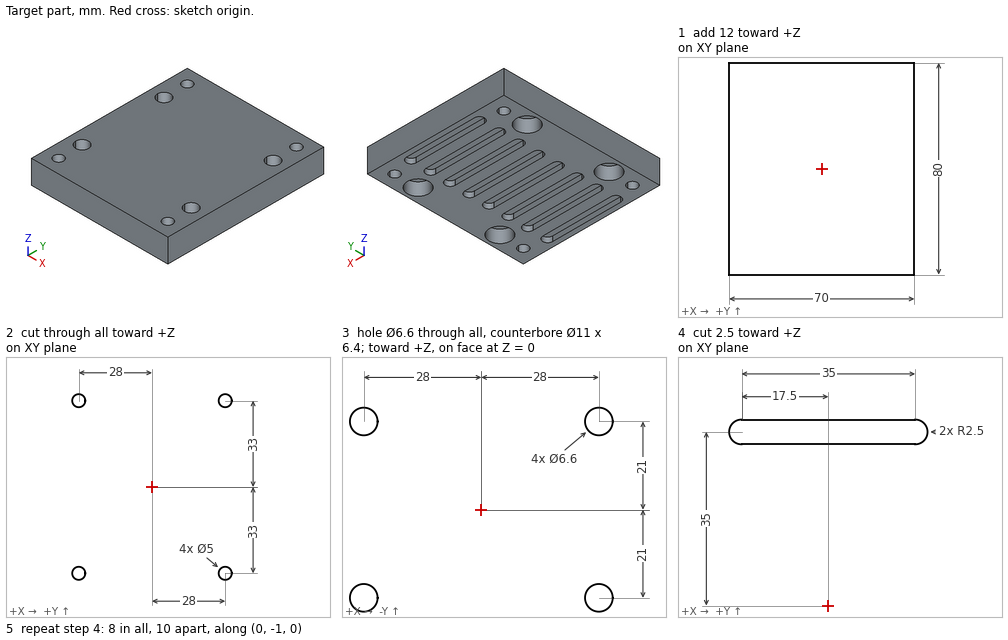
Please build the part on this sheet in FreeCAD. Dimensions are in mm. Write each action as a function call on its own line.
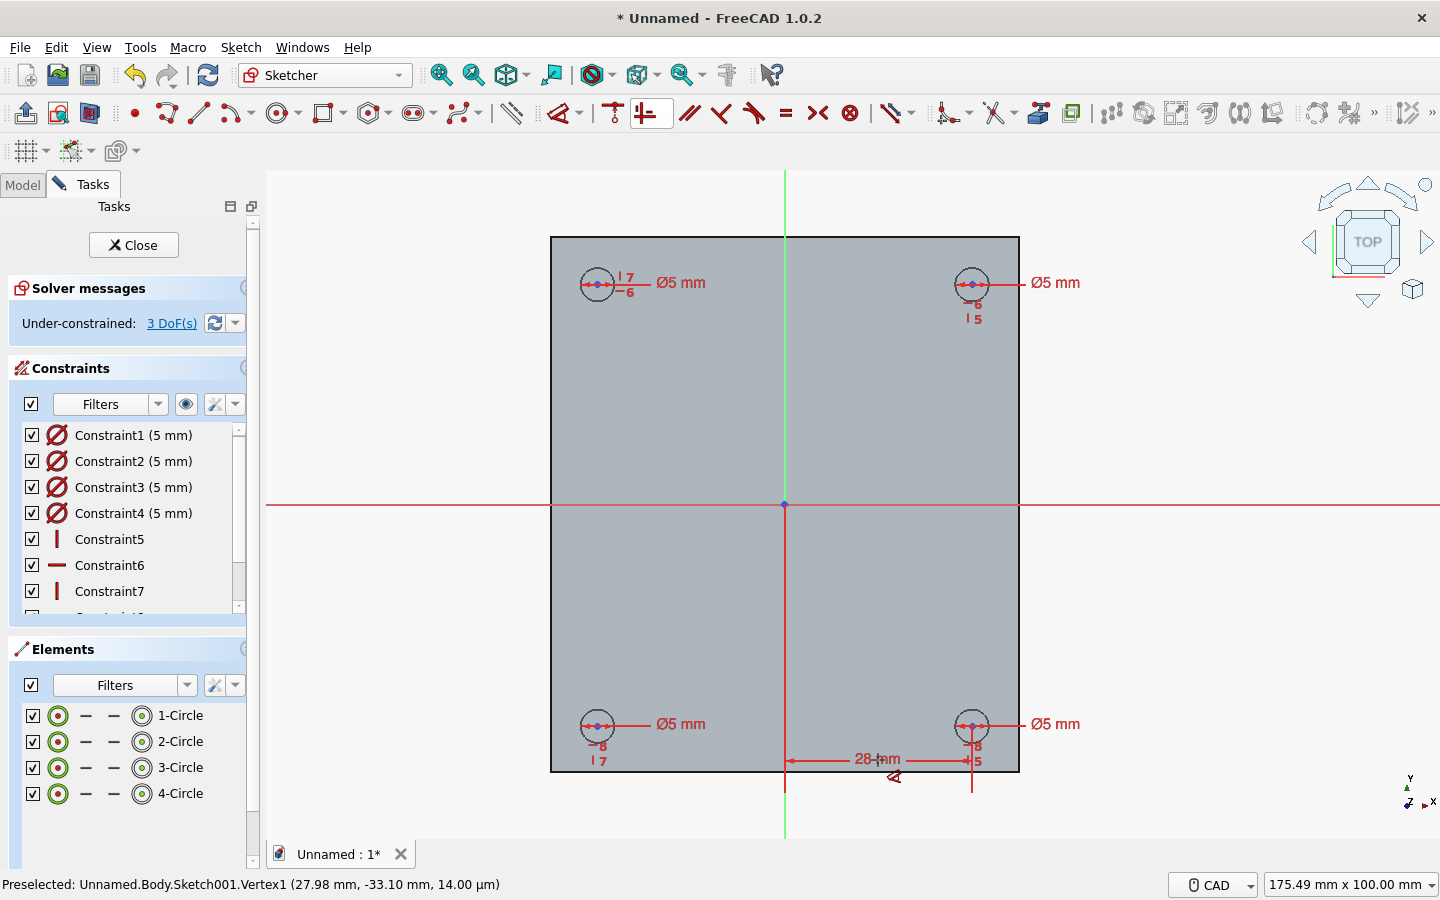
click(972, 726)
click(1006, 616)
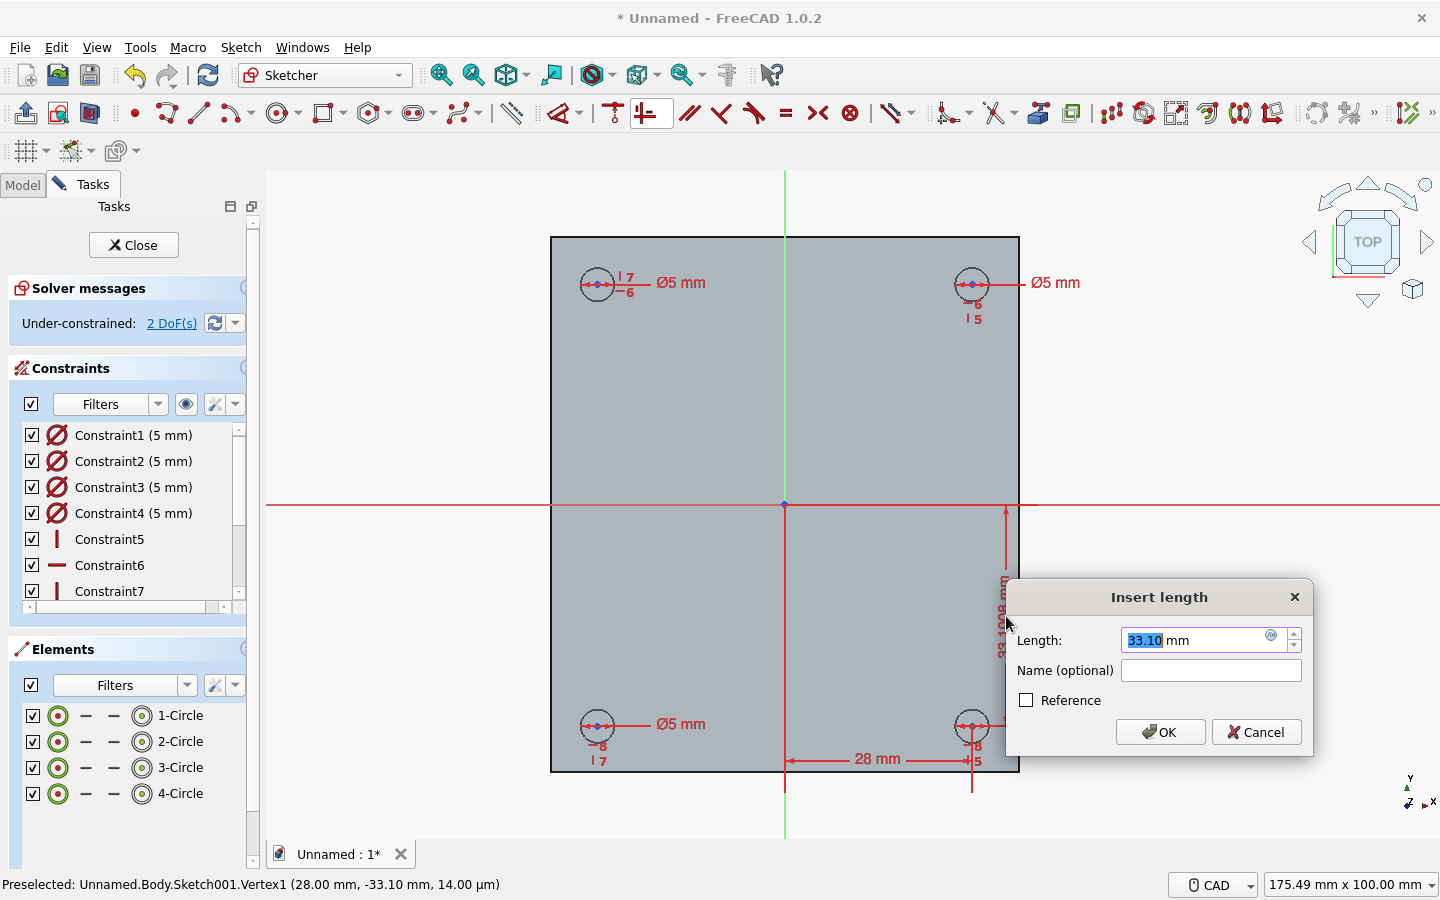
text(33)
key(Return)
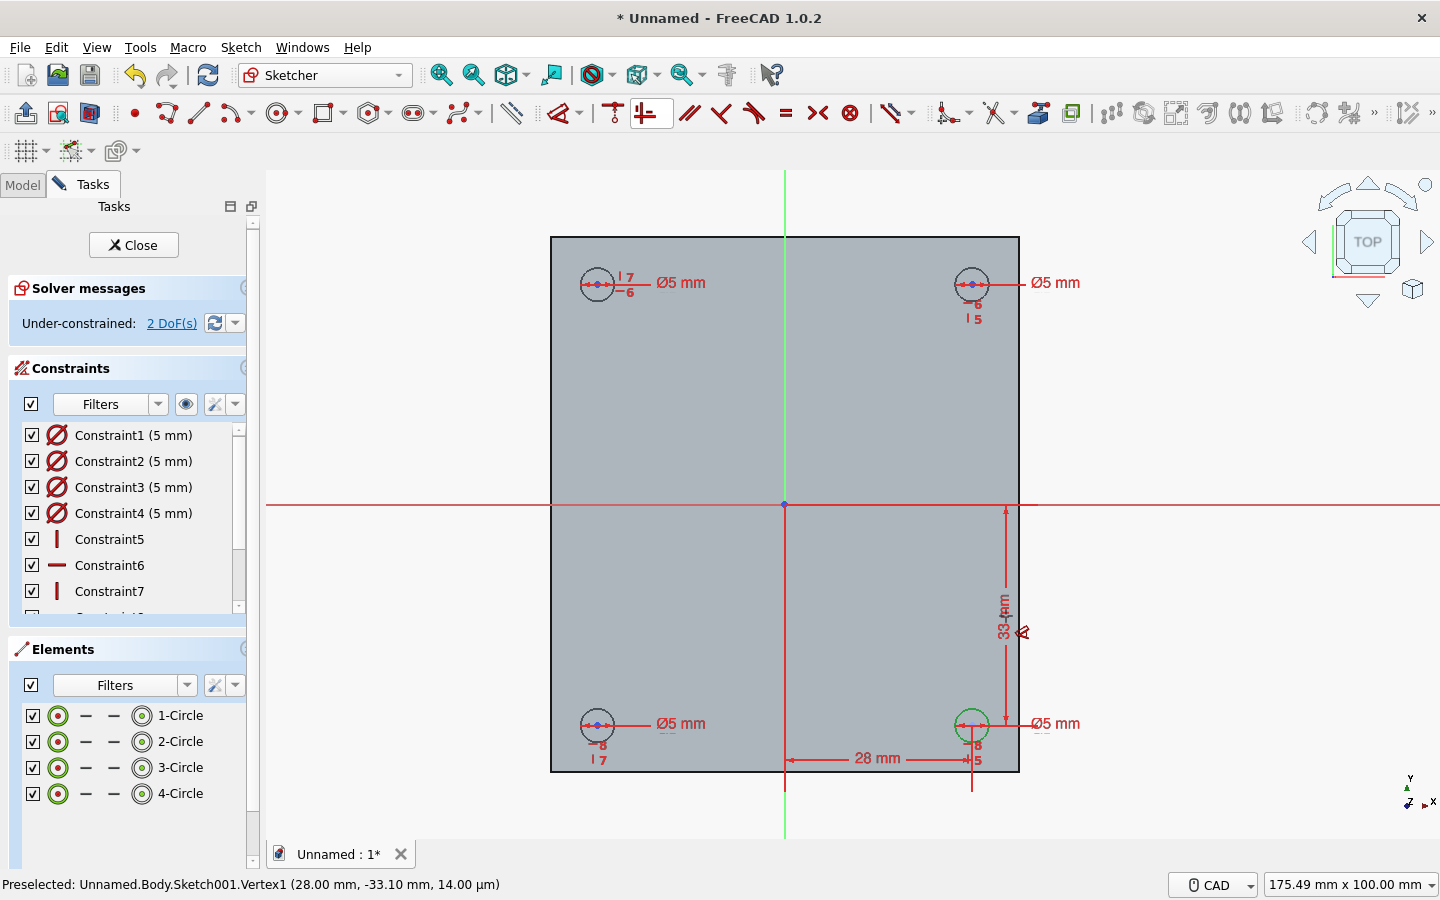
click(972, 285)
click(1006, 395)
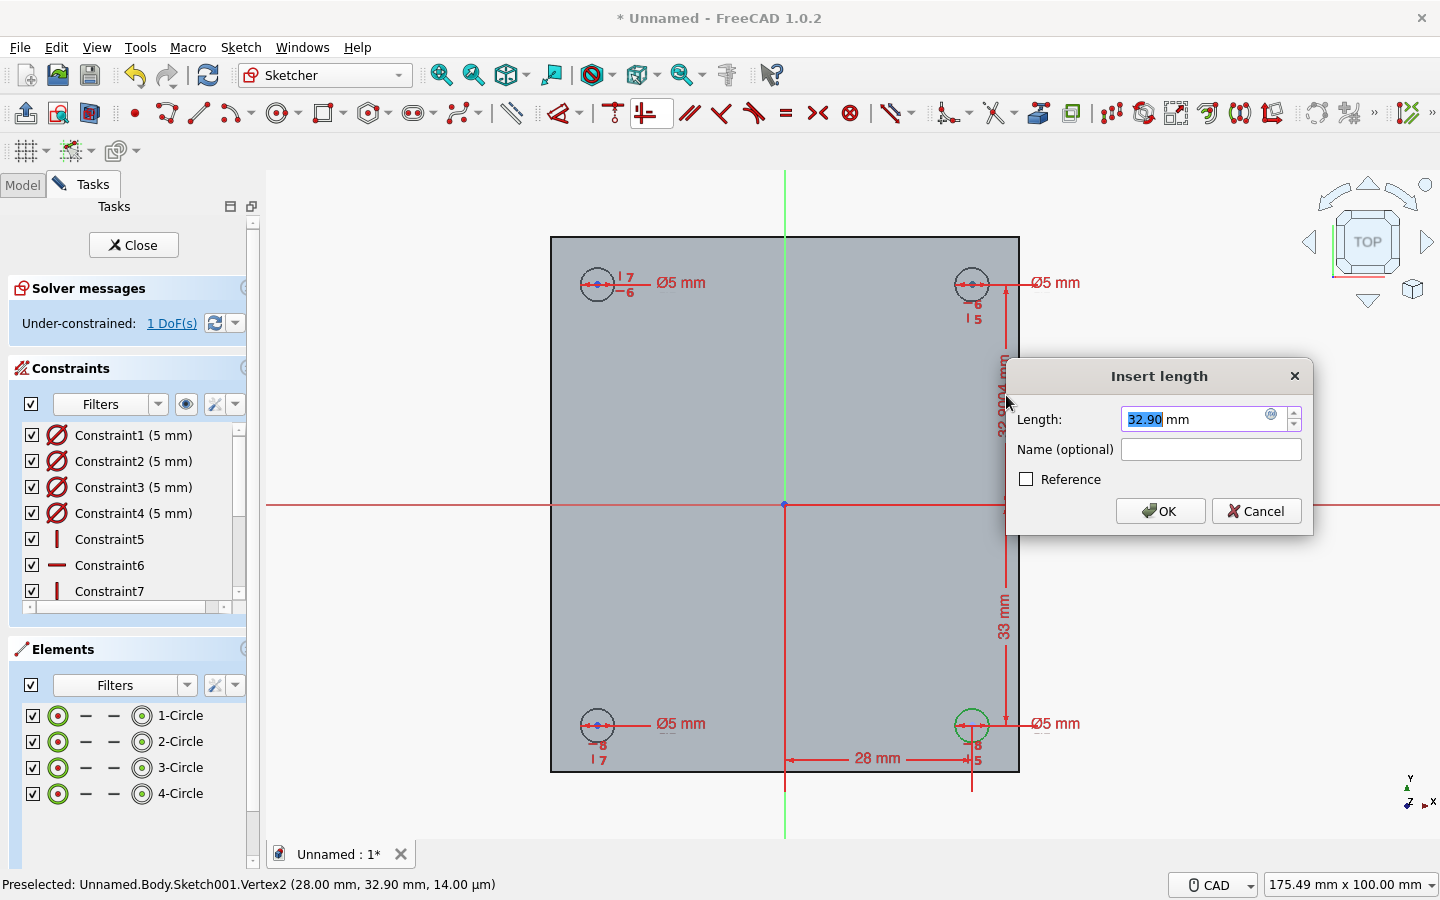
text(33)
key(Return)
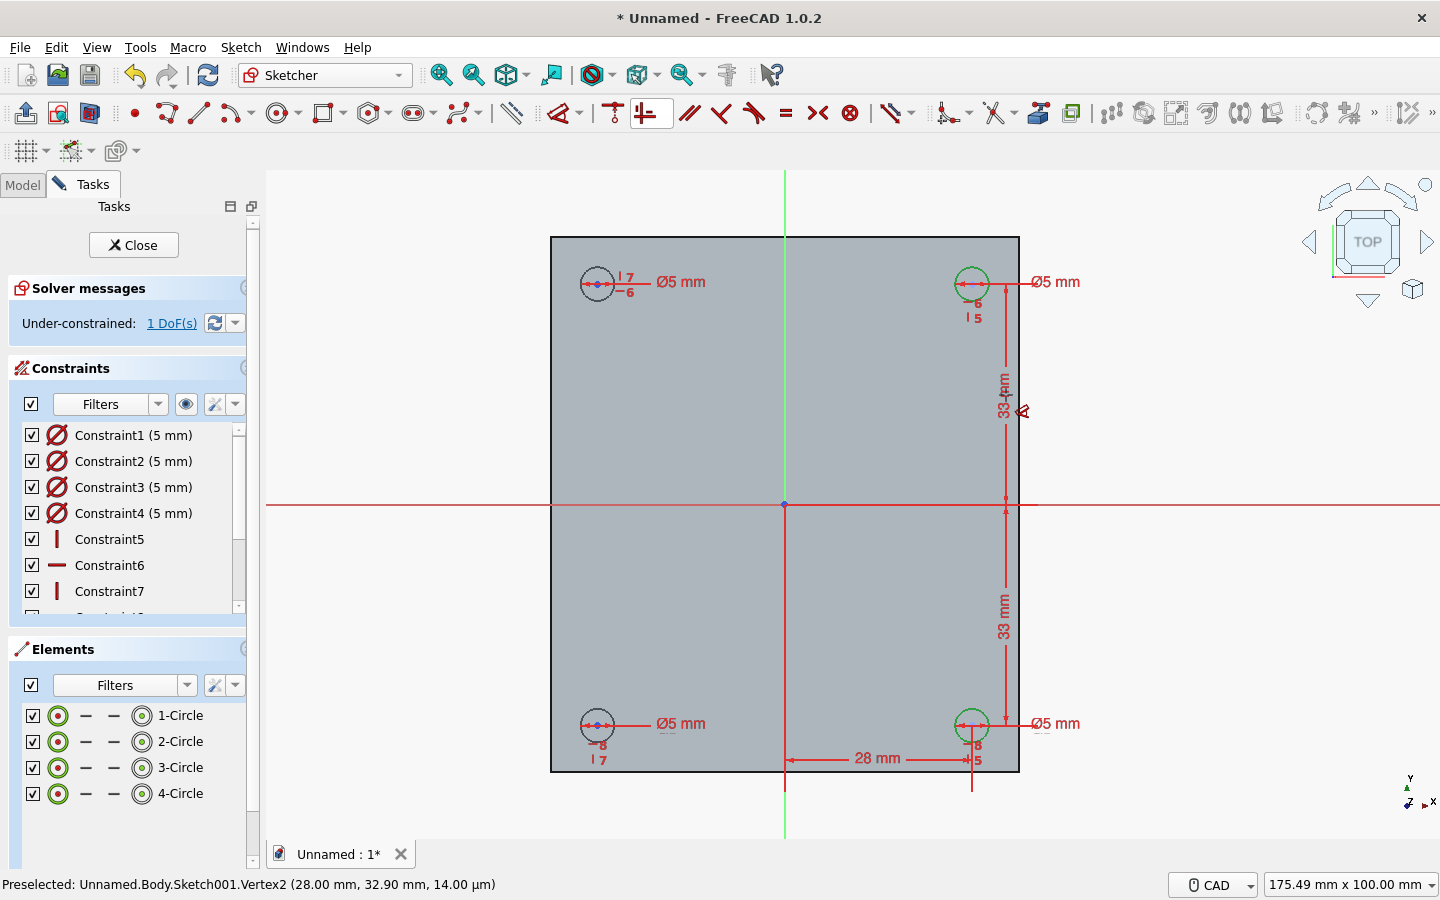
click(597, 284)
click(691, 250)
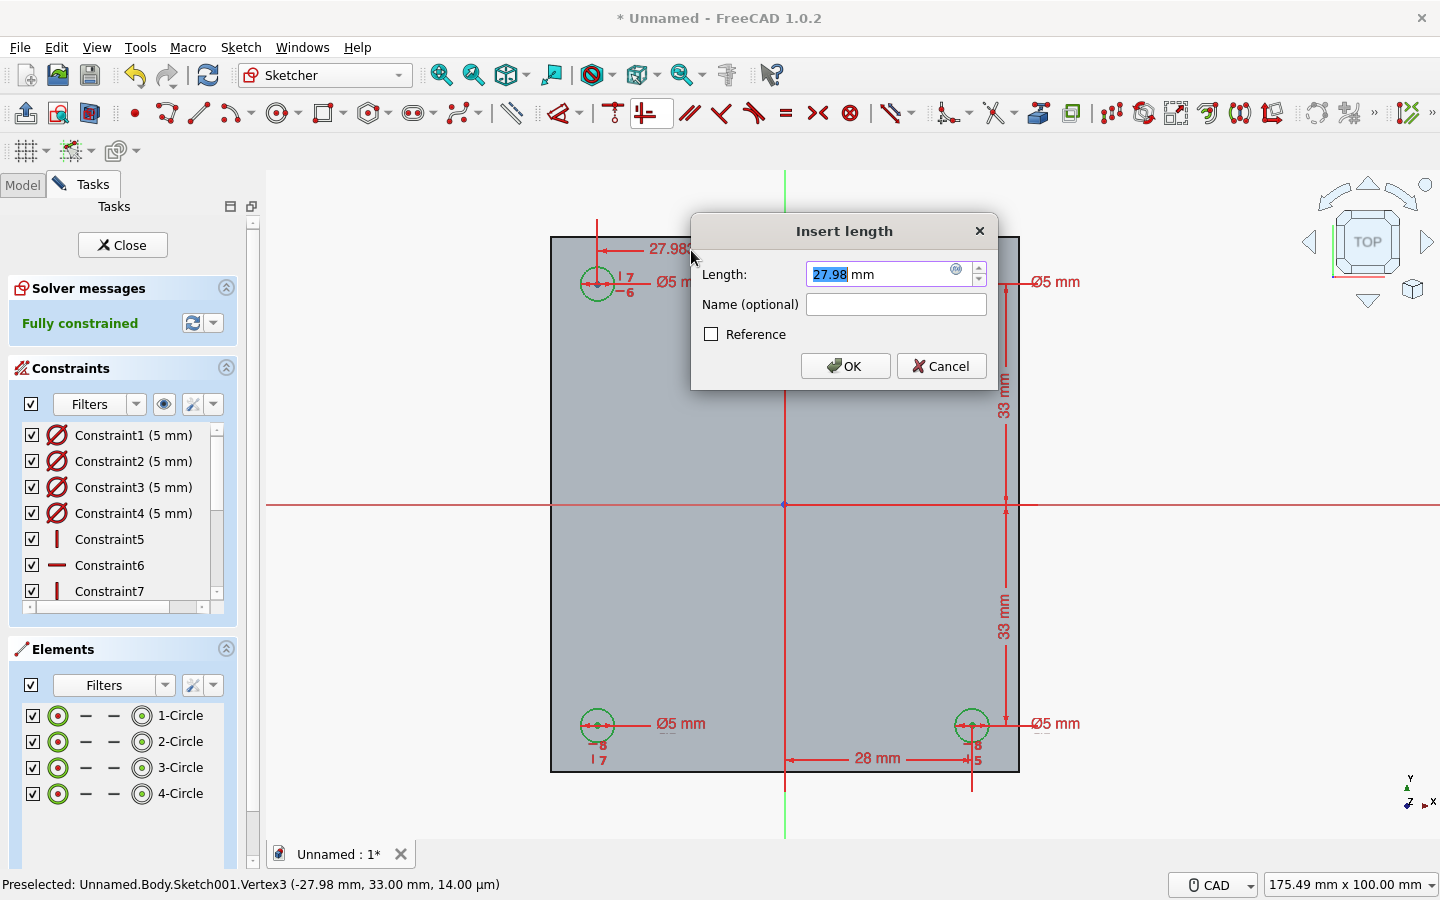
text(28)
key(Return)
key(Escape)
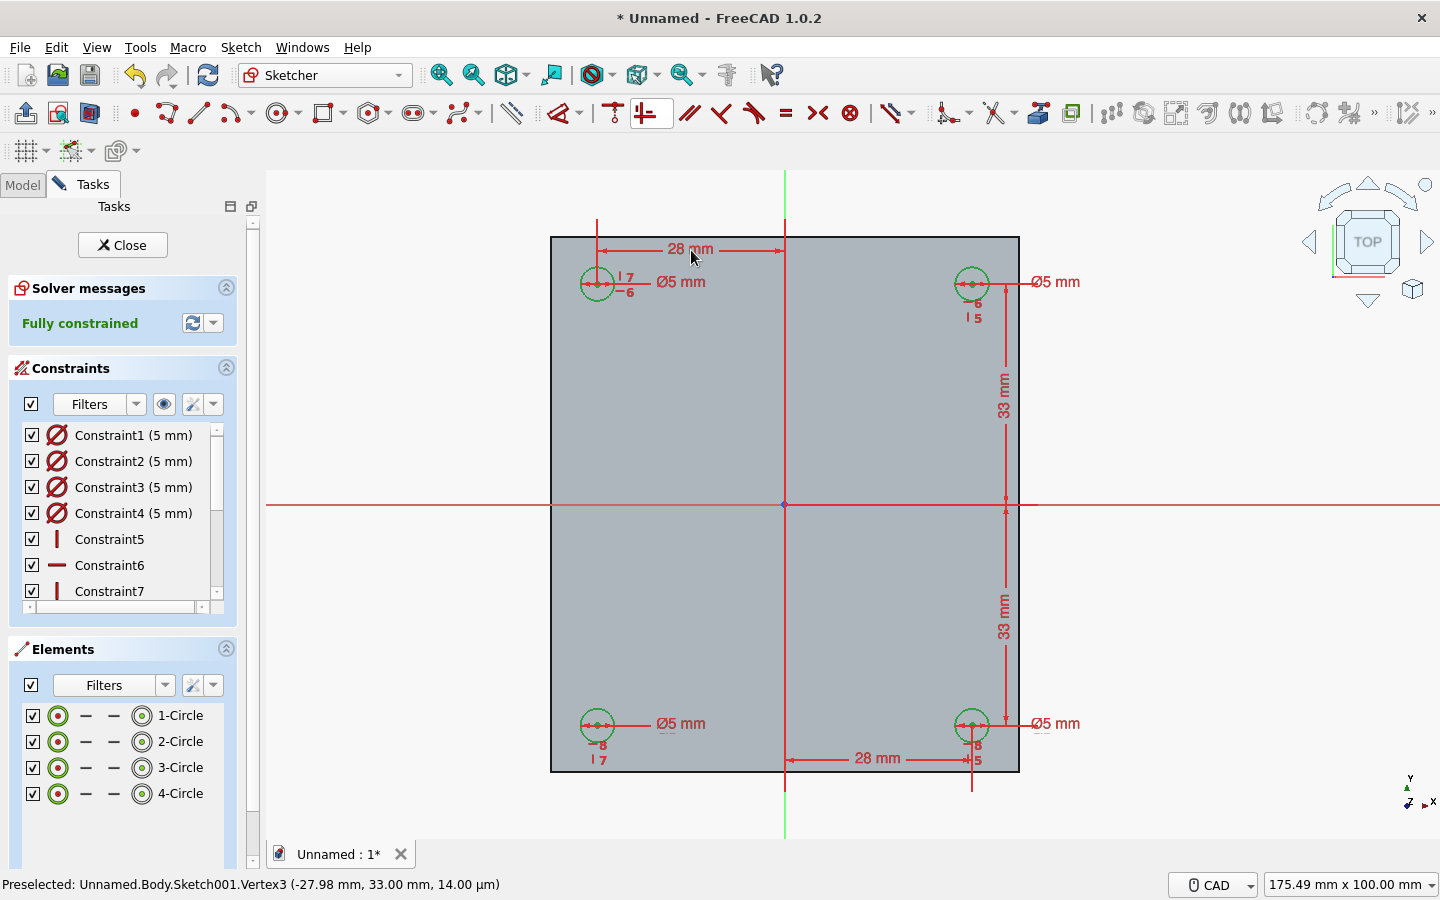
click(123, 245)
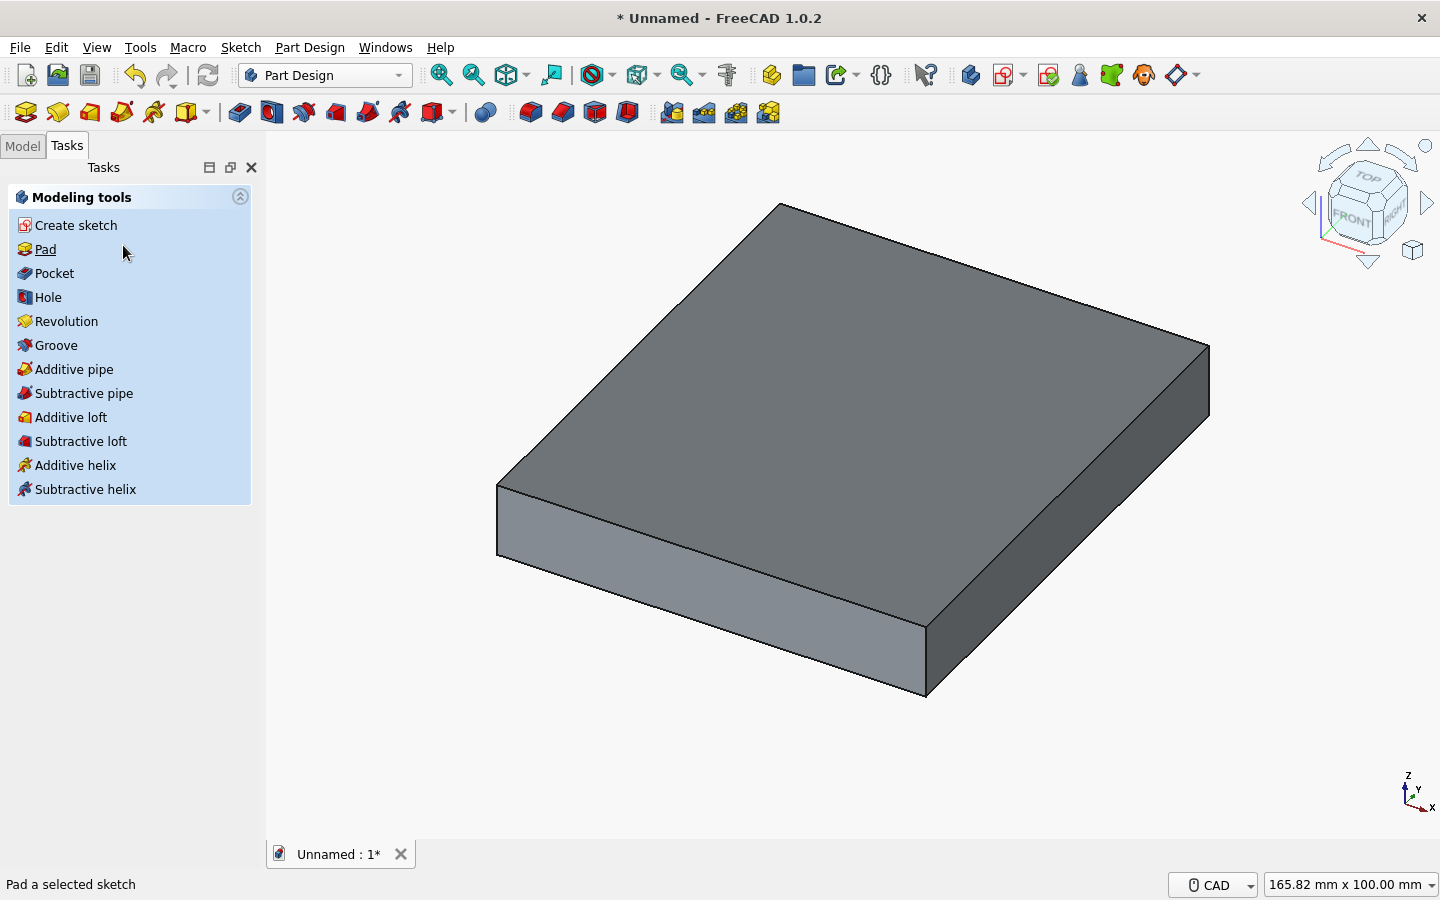
click(240, 112)